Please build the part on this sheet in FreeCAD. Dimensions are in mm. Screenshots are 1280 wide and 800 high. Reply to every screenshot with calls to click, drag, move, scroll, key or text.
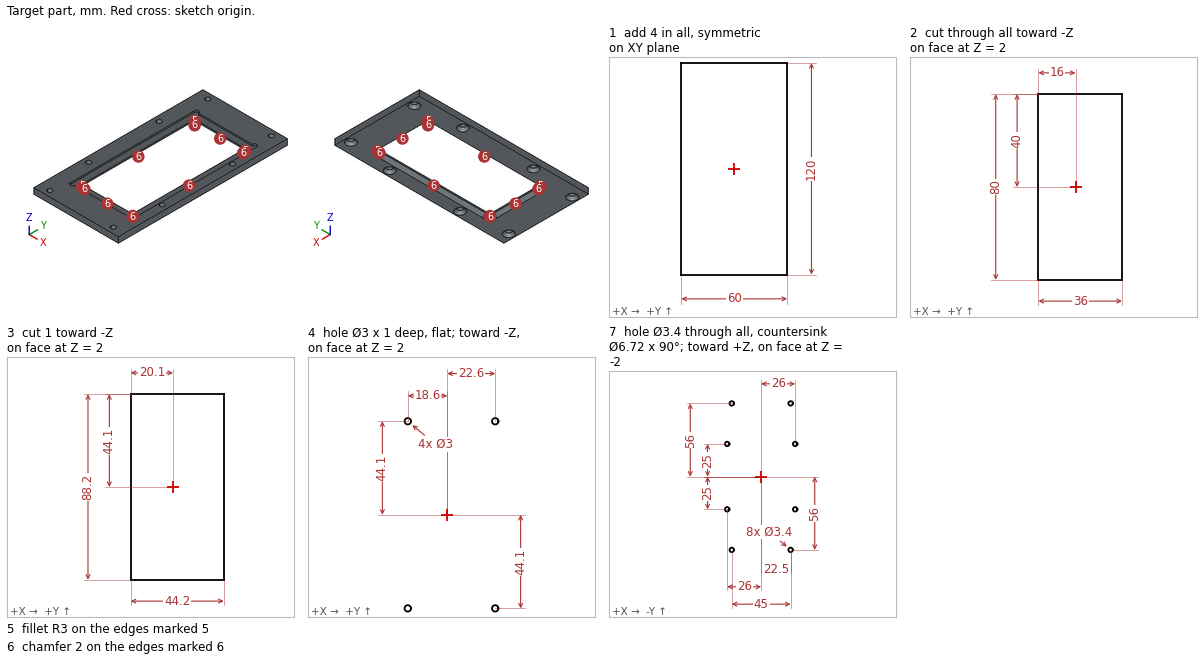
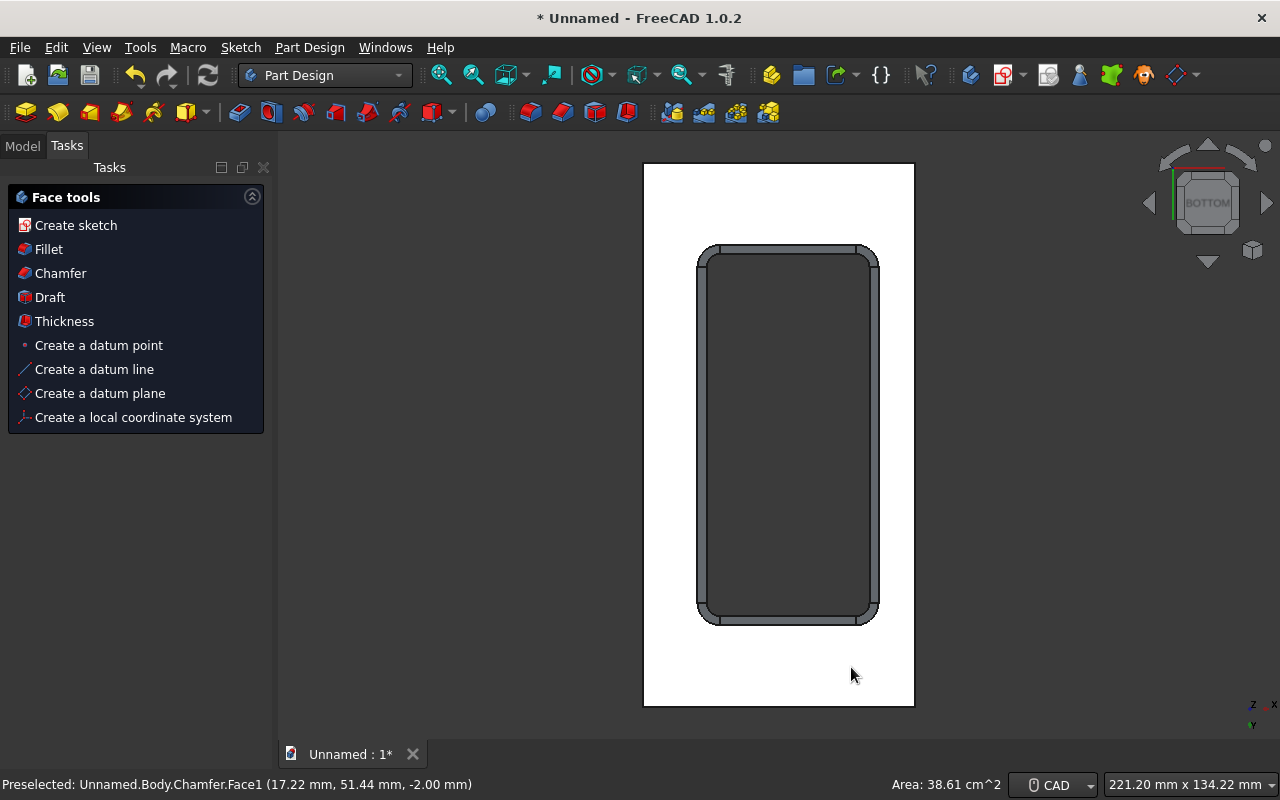
click(1004, 76)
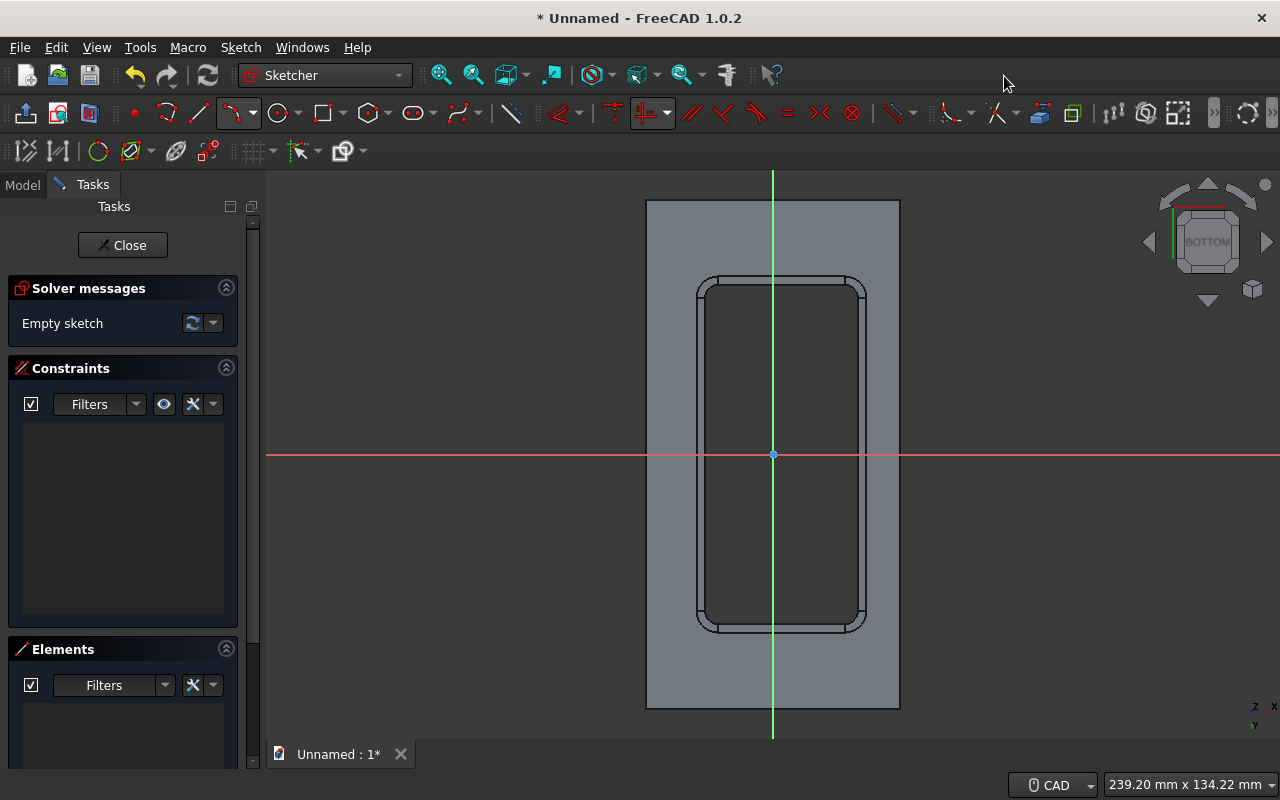
scroll(565, 455, down, 2)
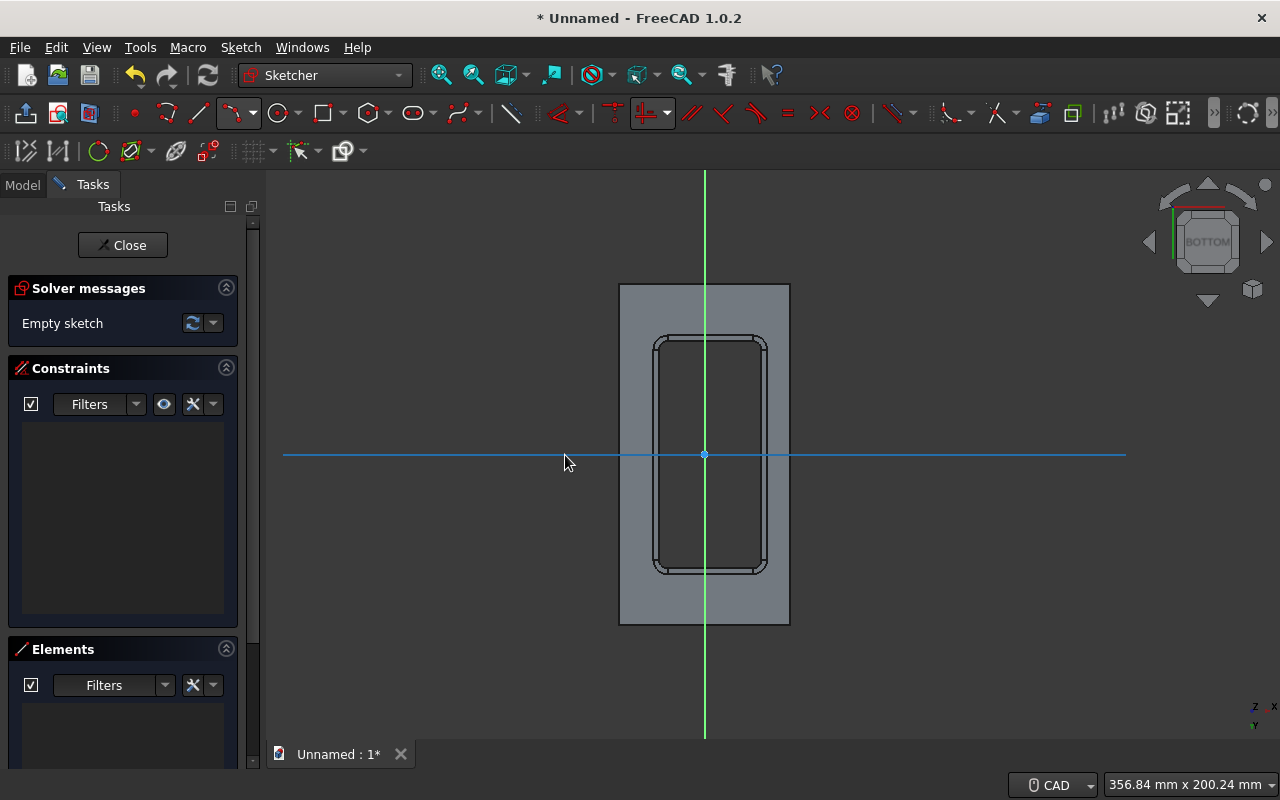
click(278, 114)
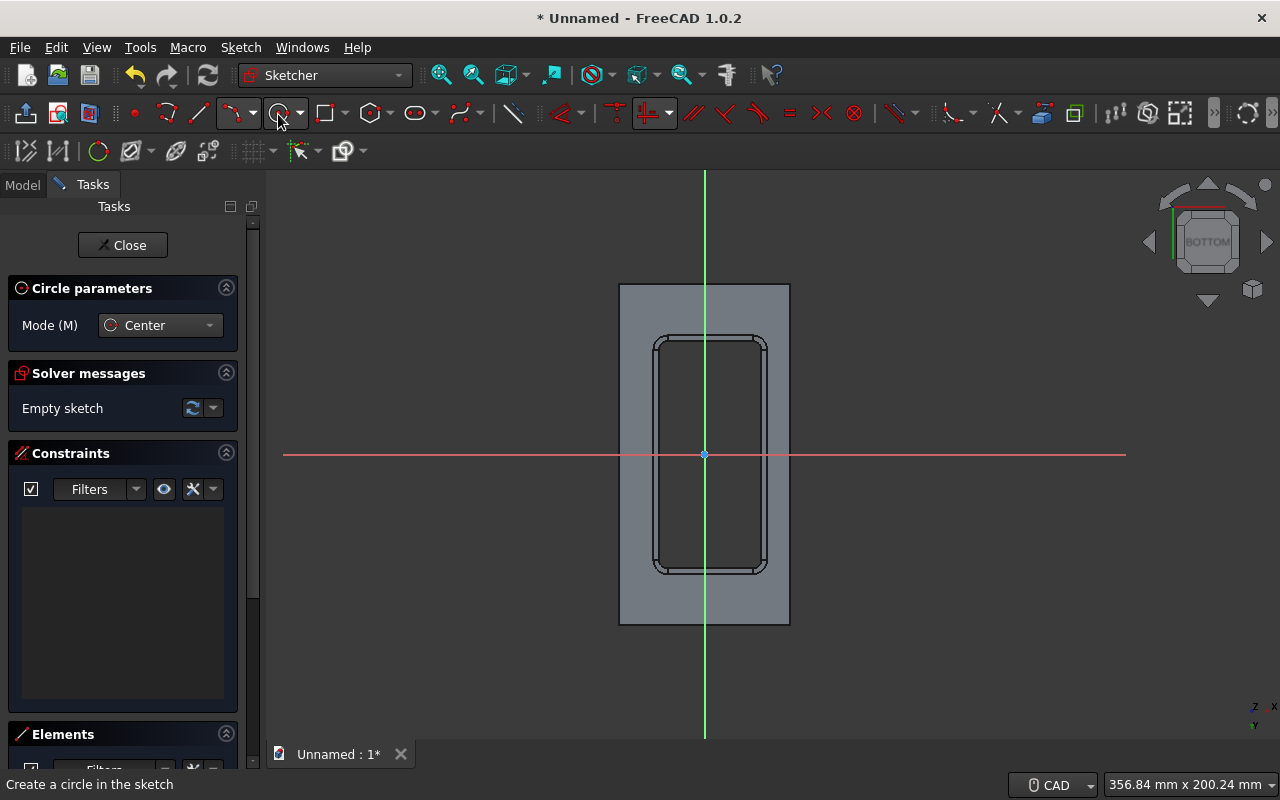
scroll(768, 614, up, 8)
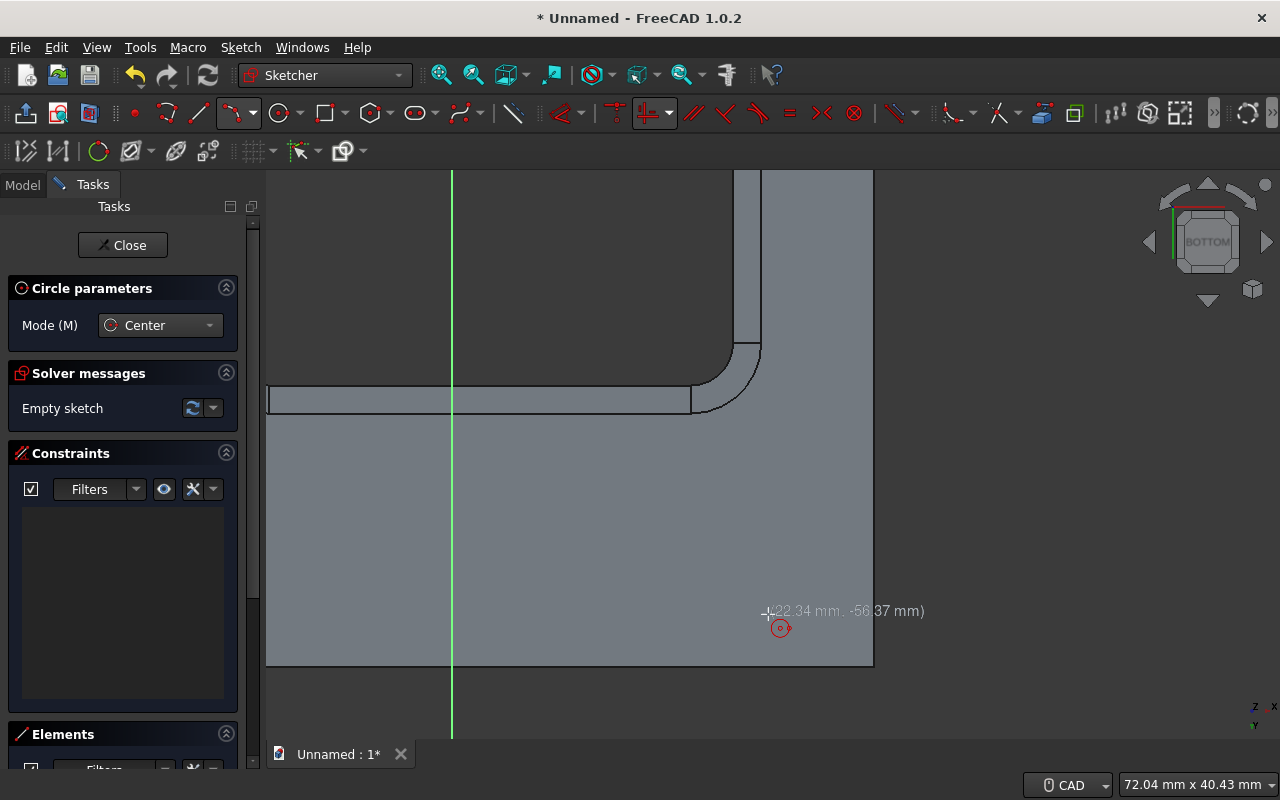
scroll(768, 614, down, 8)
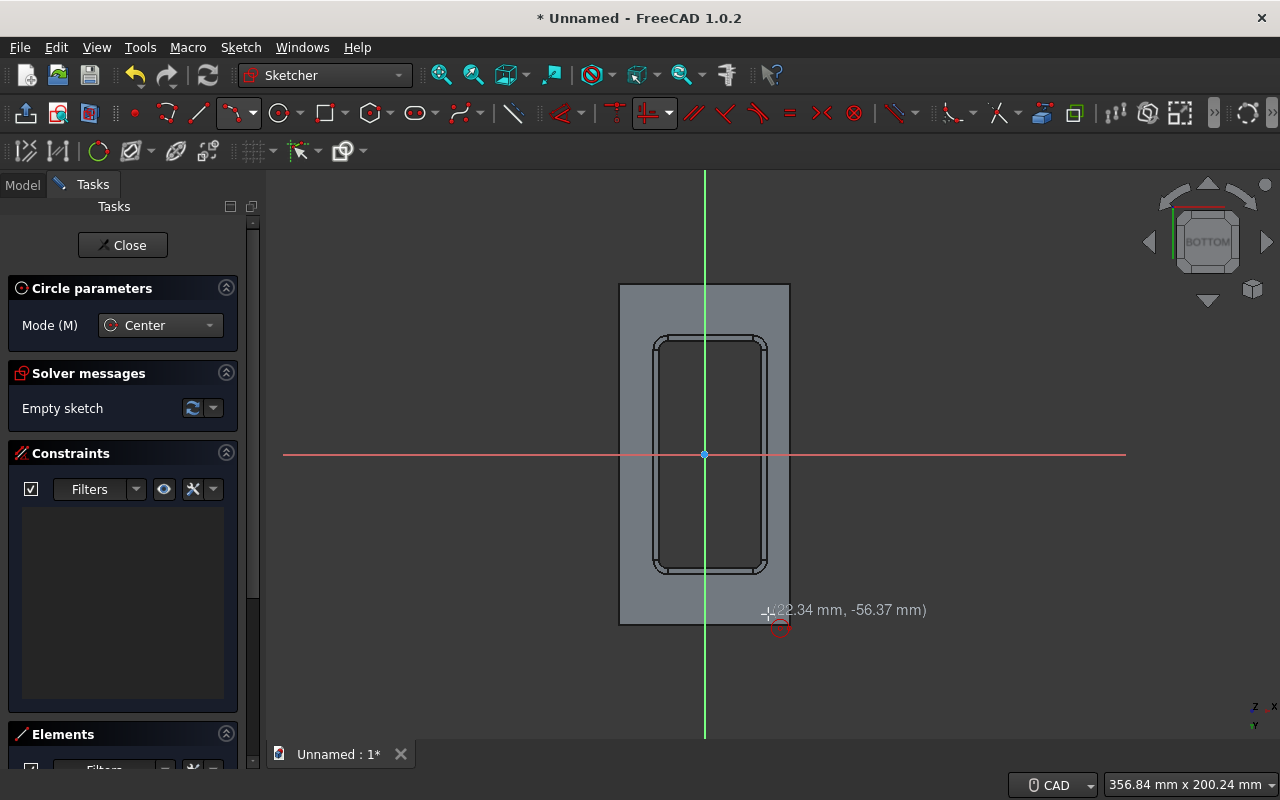
click(768, 614)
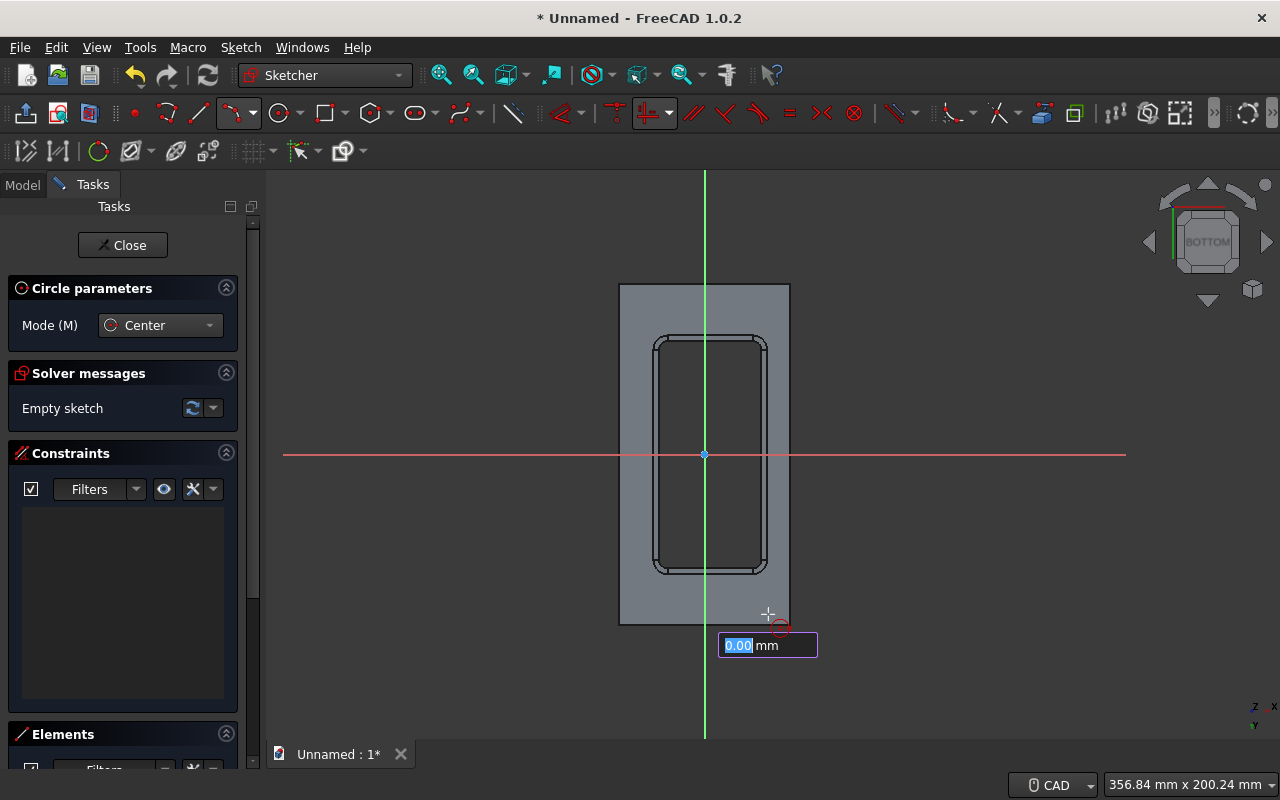
scroll(772, 611, up, 6)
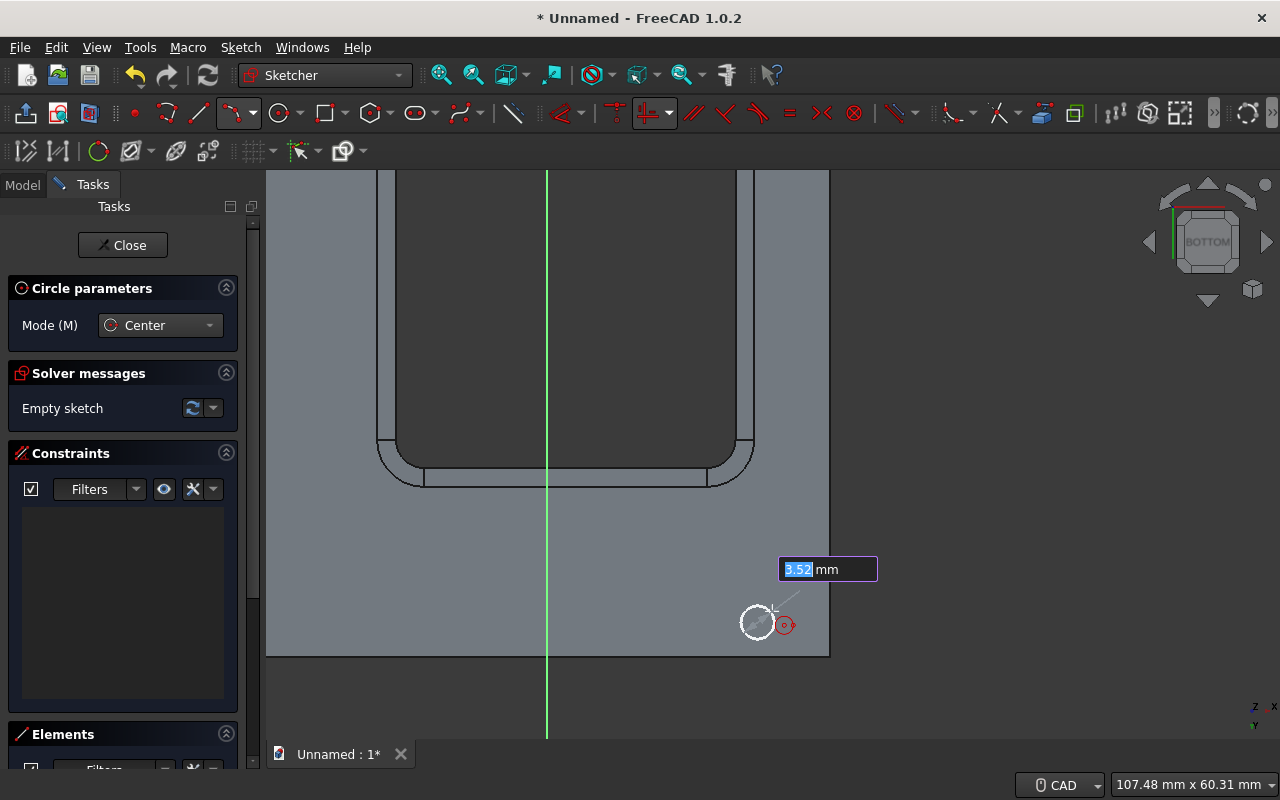
click(770, 608)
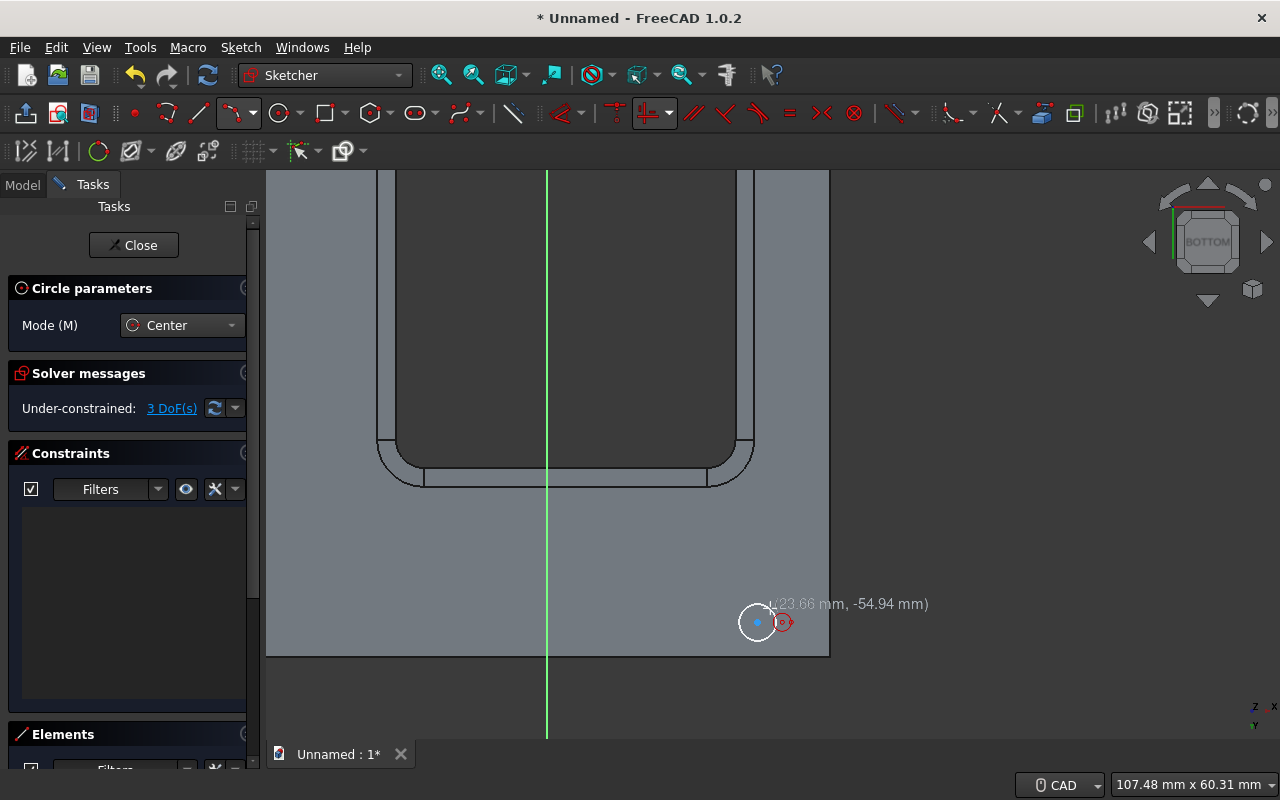
scroll(335, 619, up, 2)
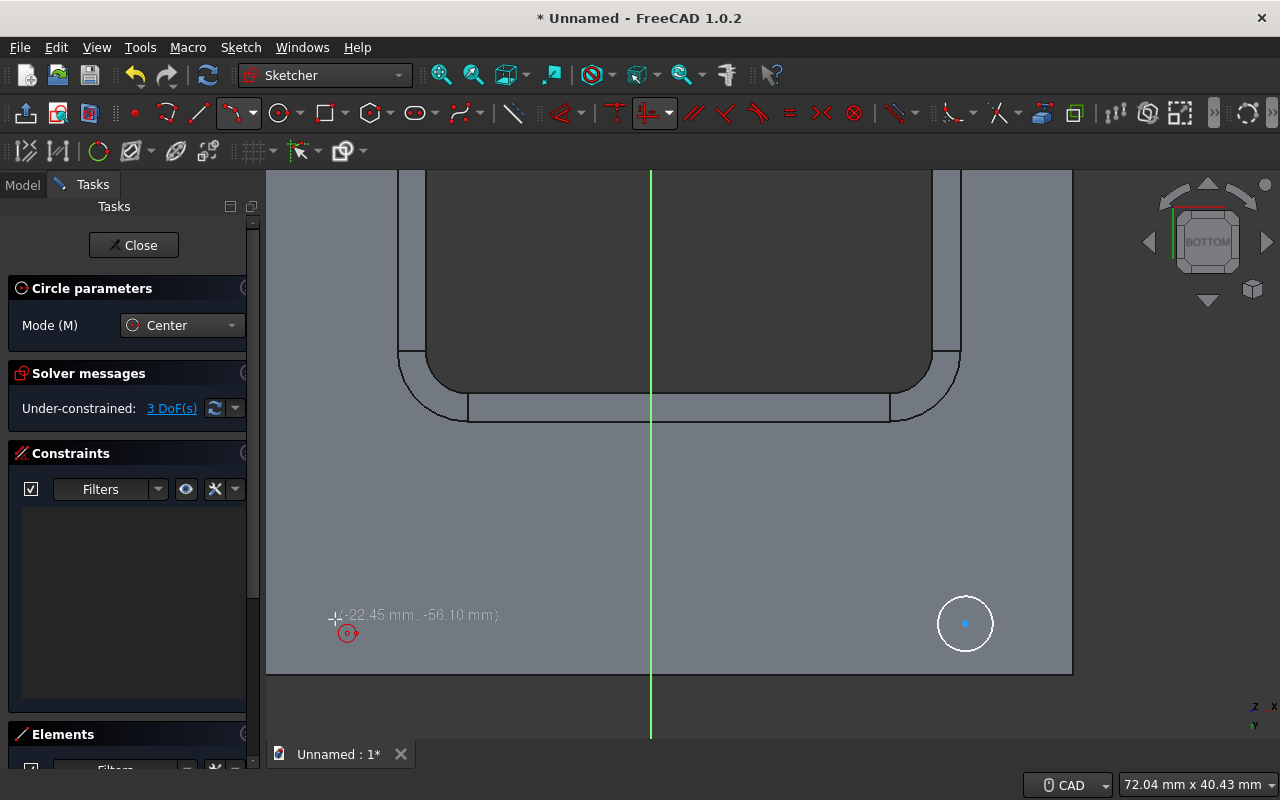
scroll(718, 612, down, 8)